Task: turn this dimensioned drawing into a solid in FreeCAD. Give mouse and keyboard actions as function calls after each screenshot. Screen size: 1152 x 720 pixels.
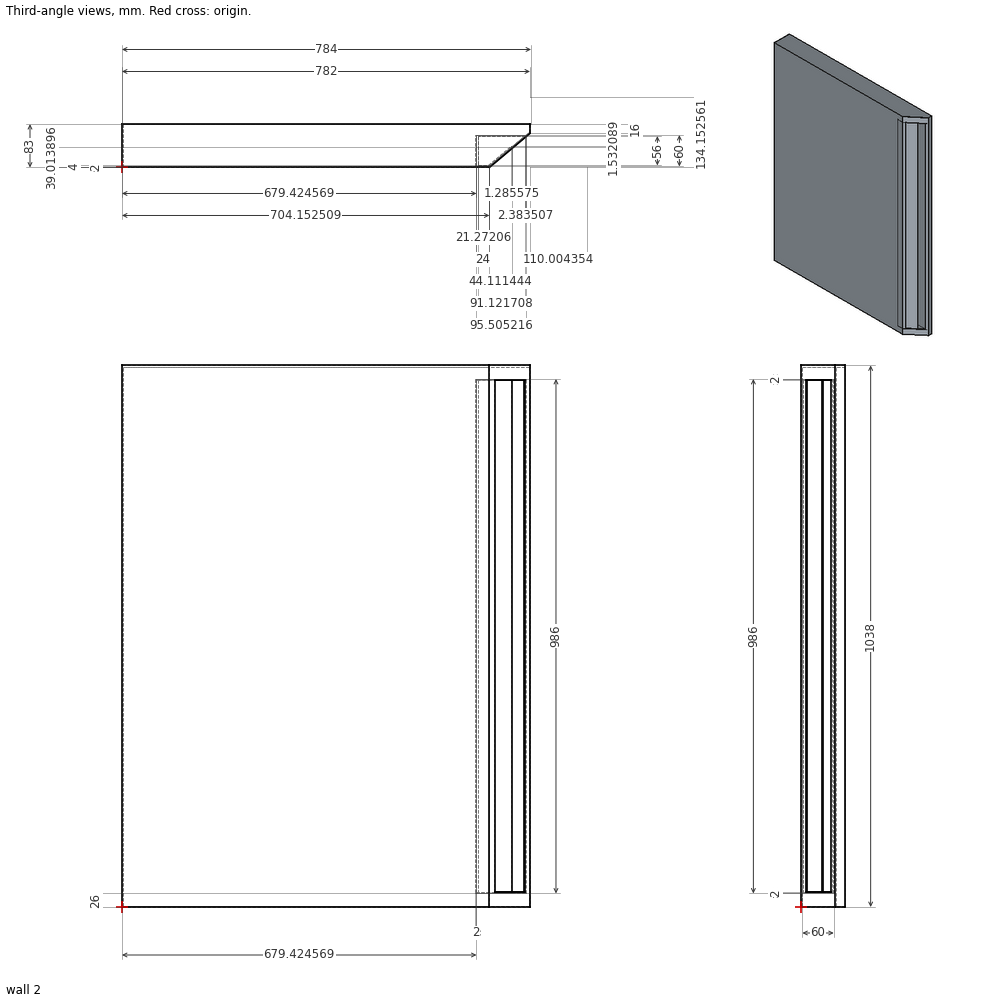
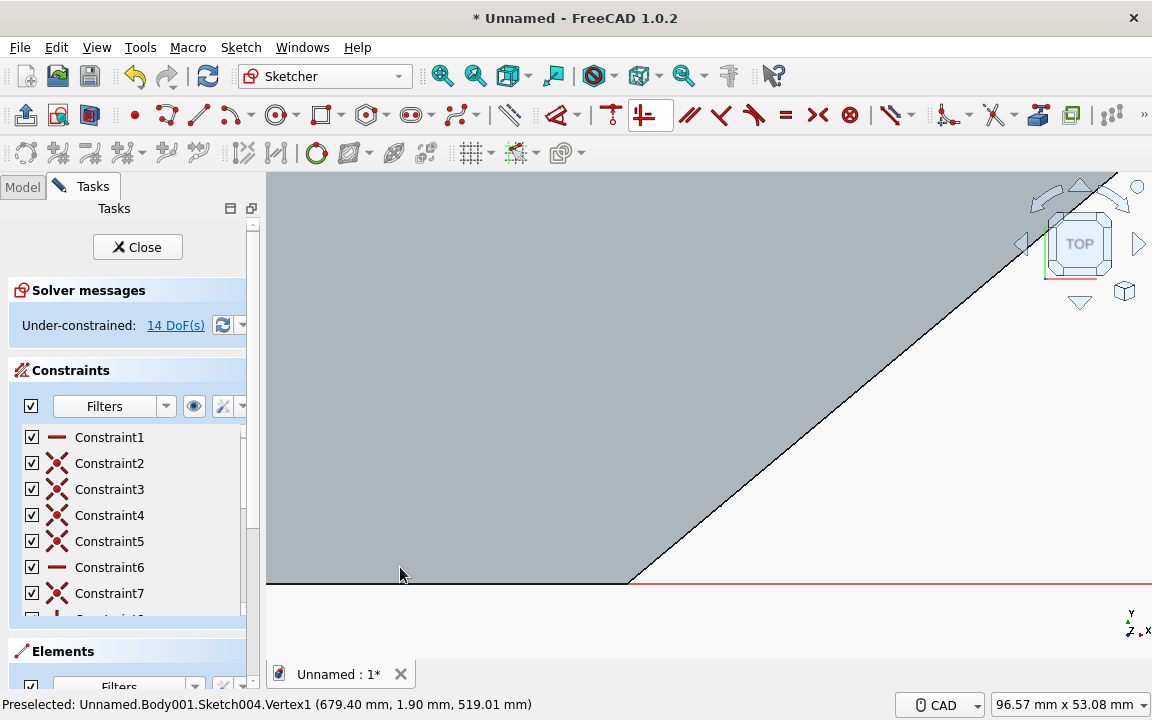
click(556, 116)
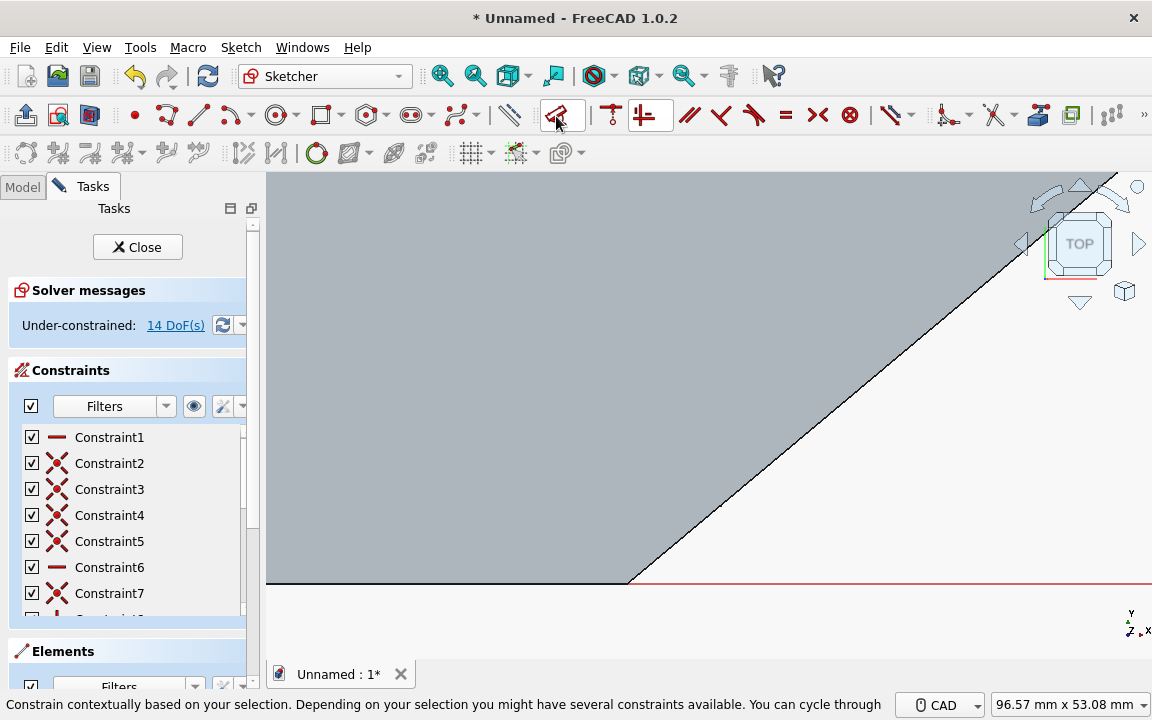
click(466, 567)
click(510, 601)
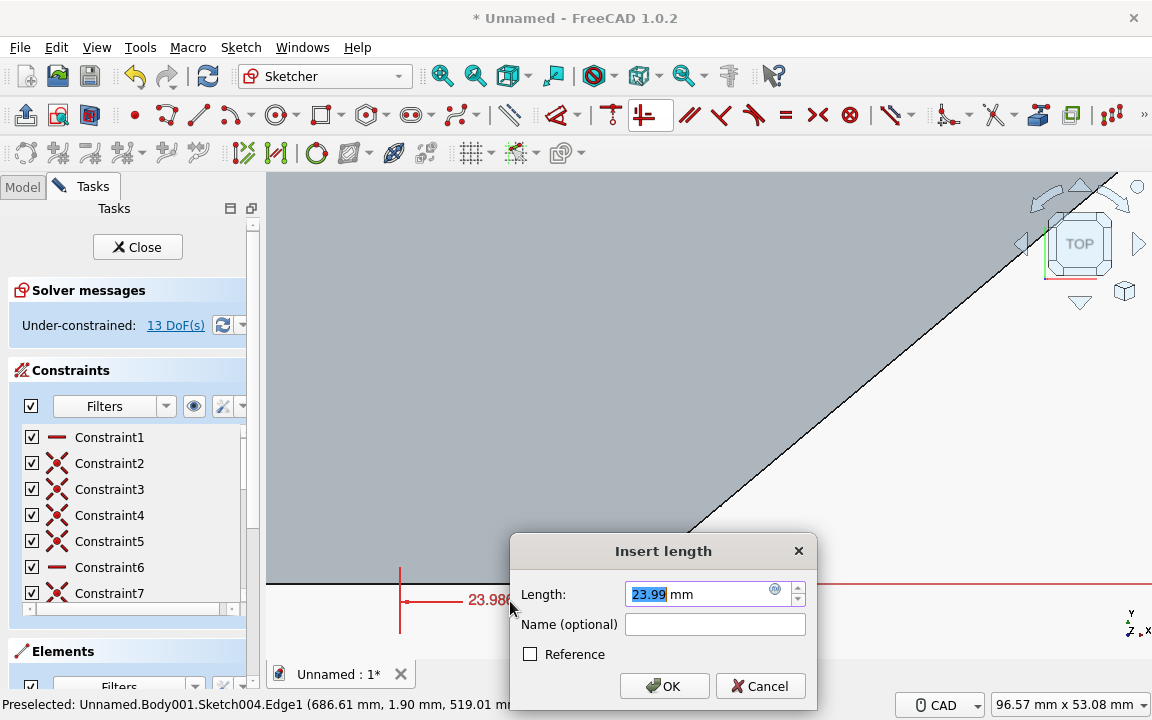
text(24)
key(Return)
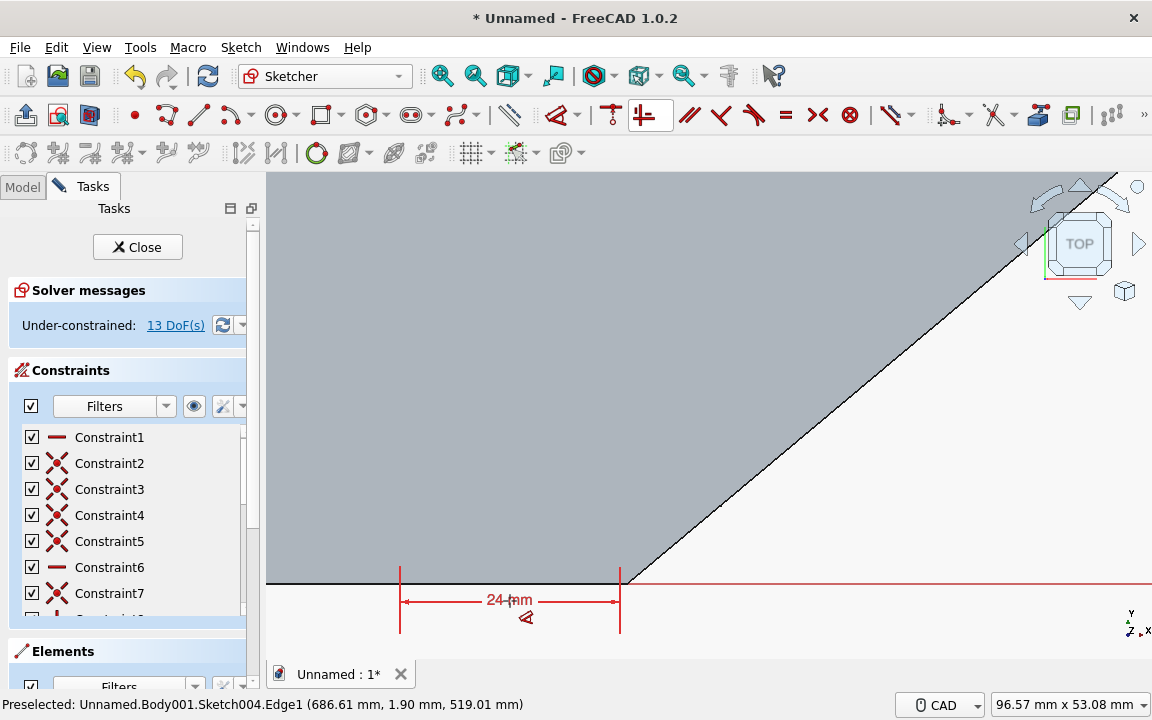
click(418, 395)
click(384, 374)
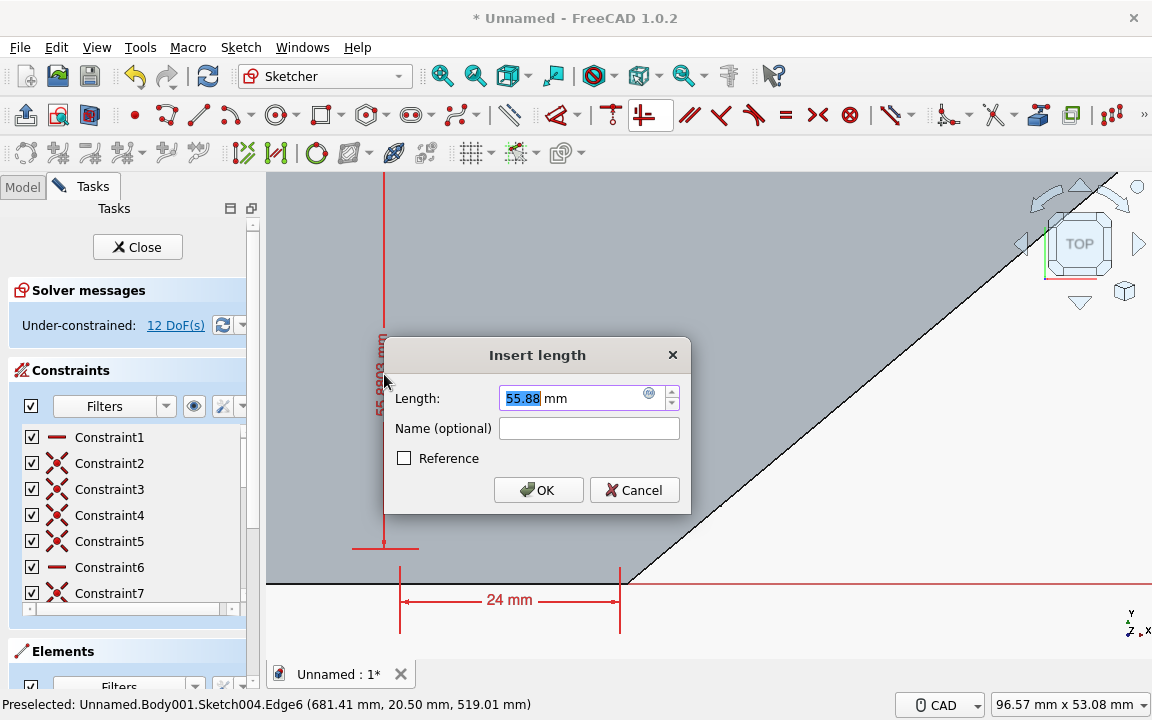
text(56)
key(Return)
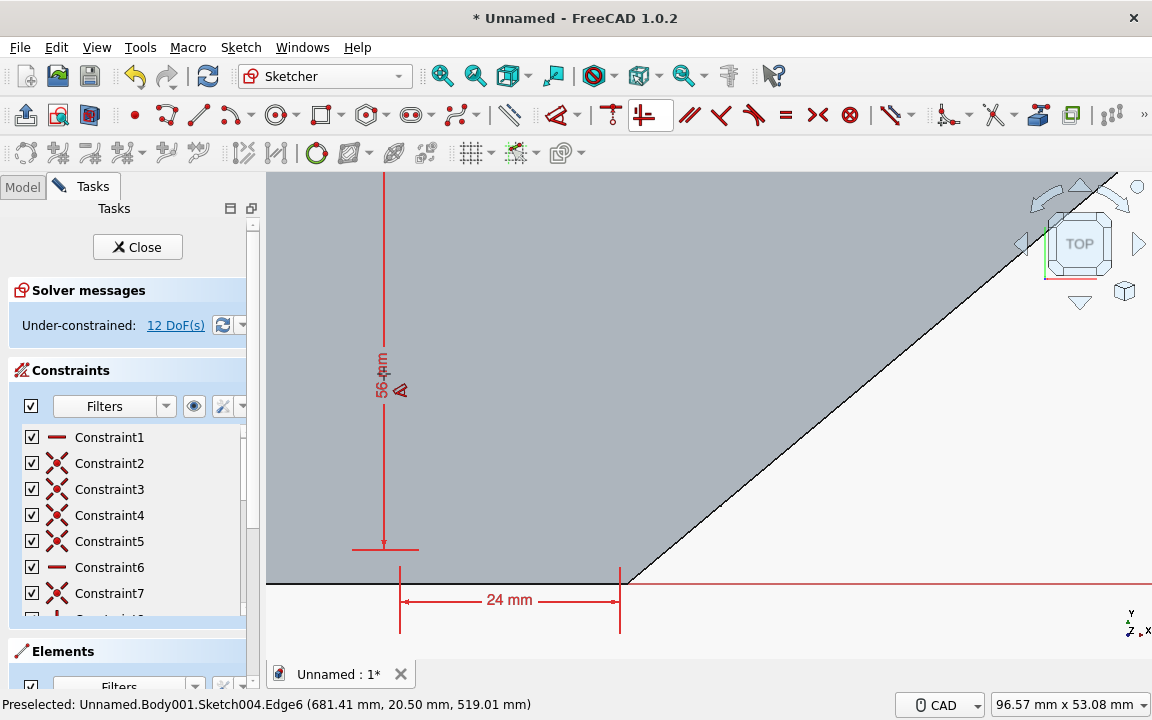
click(400, 402)
click(366, 299)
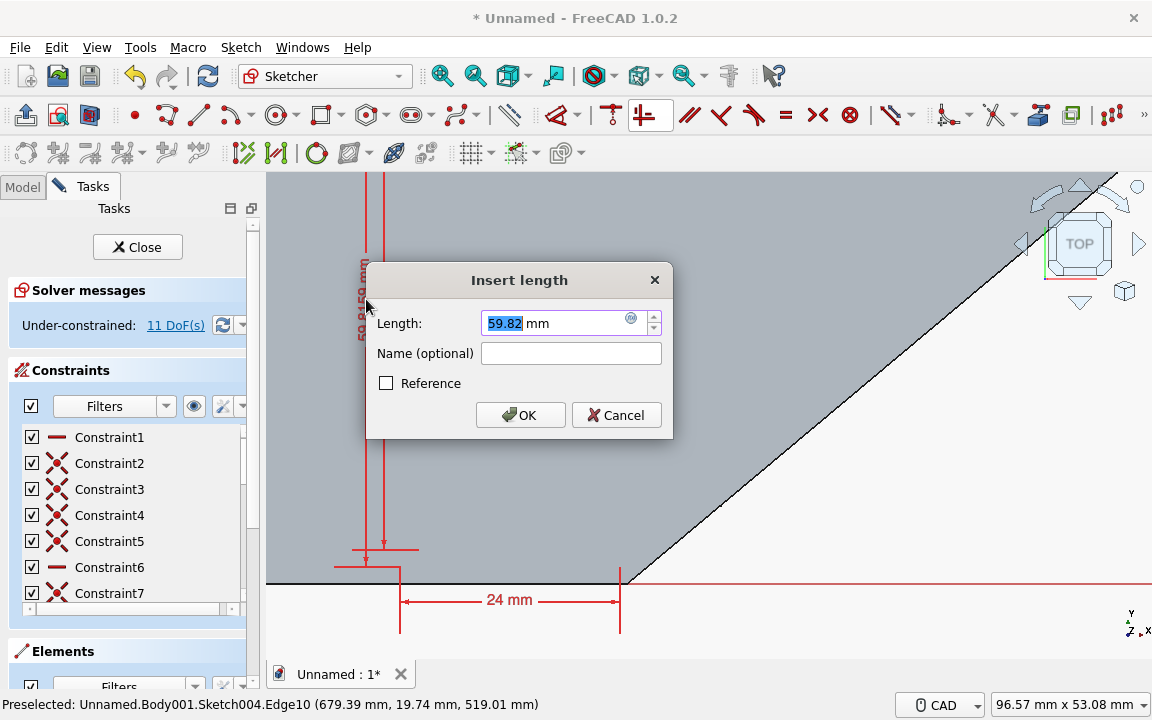
text(60)
key(Return)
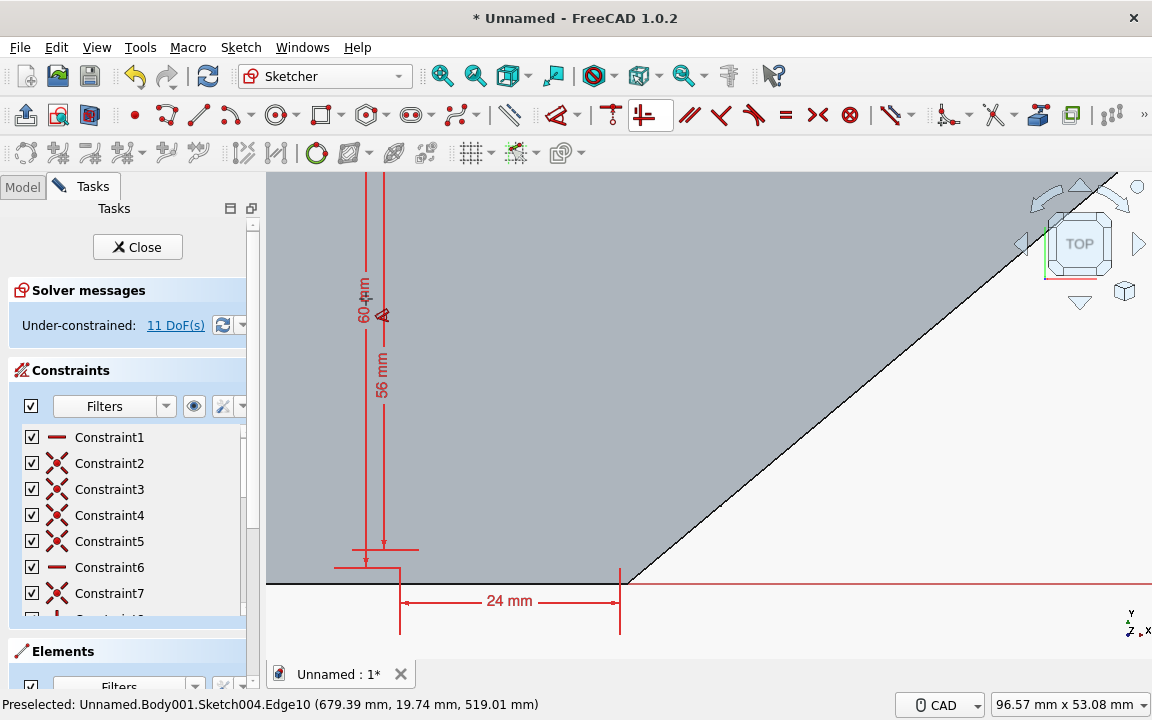
scroll(400, 568, up, 4)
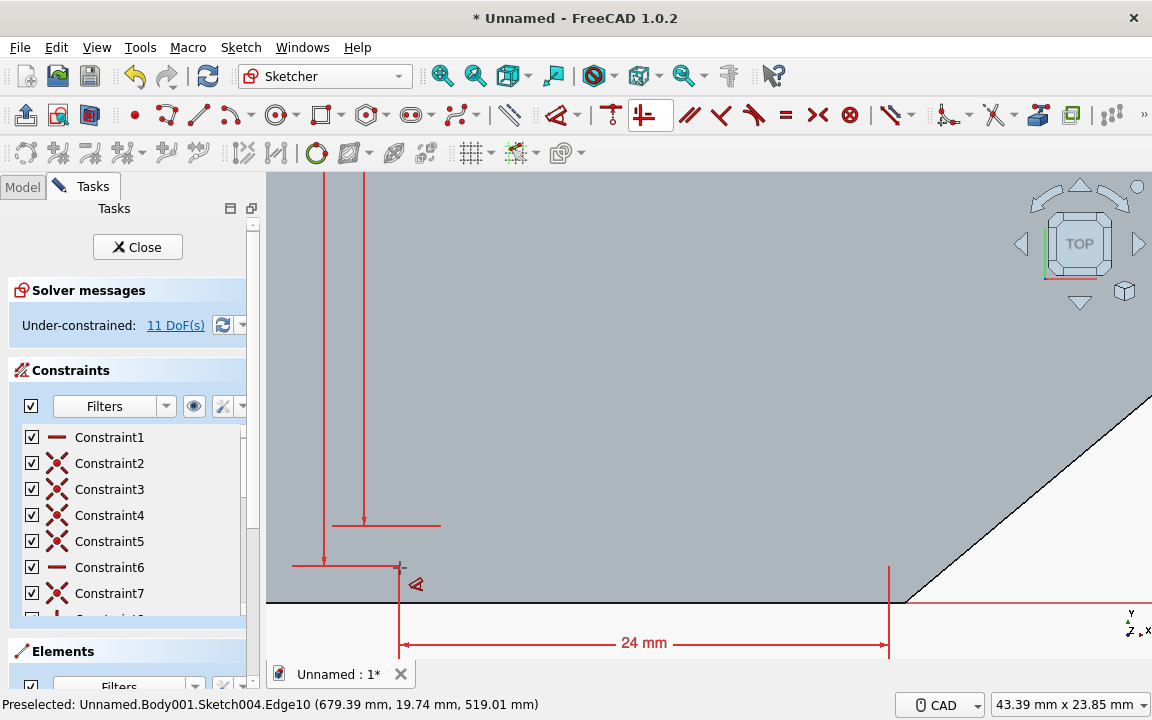
click(399, 566)
click(433, 585)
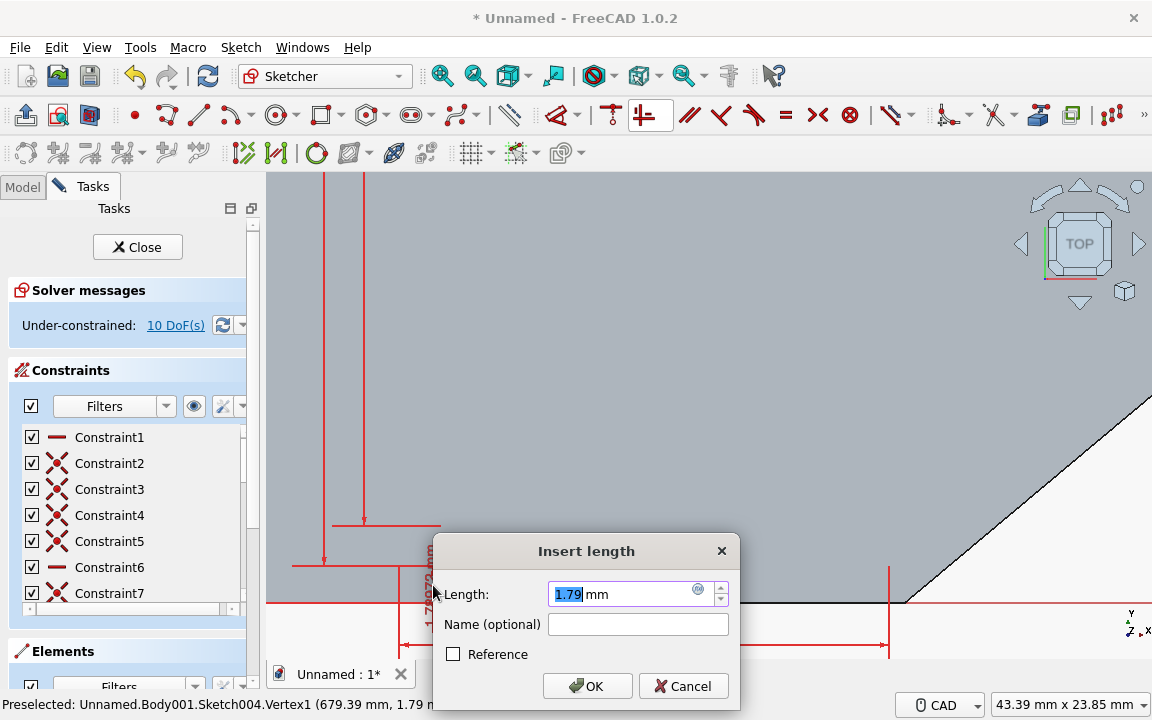
text(2)
key(Return)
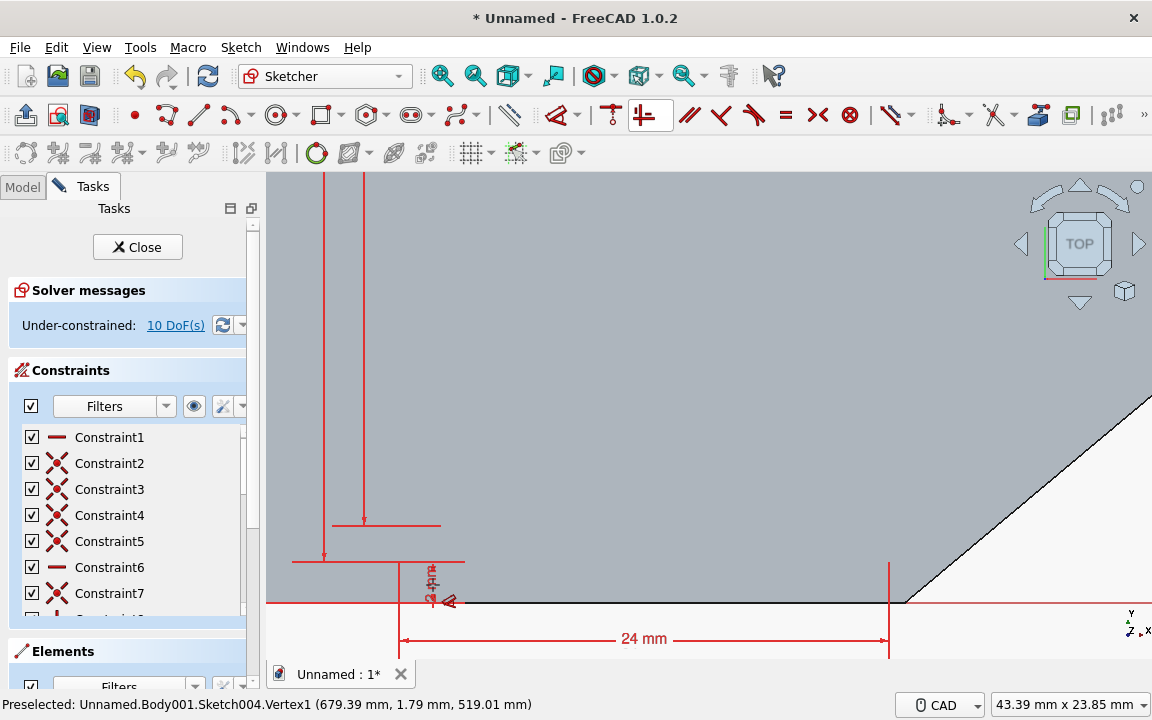
click(875, 526)
click(909, 565)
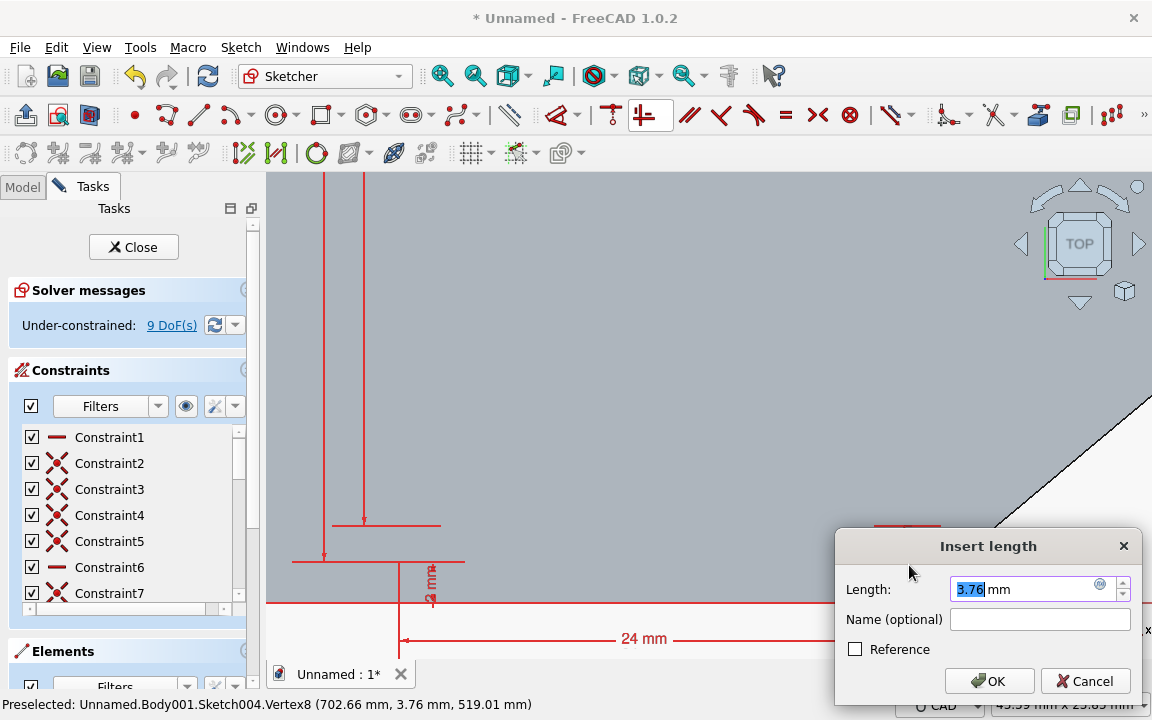
text(4)
key(Return)